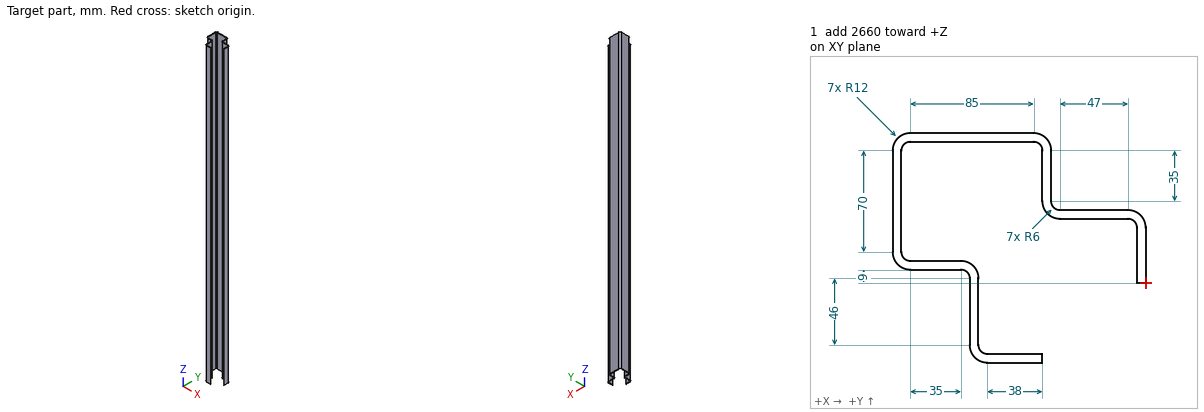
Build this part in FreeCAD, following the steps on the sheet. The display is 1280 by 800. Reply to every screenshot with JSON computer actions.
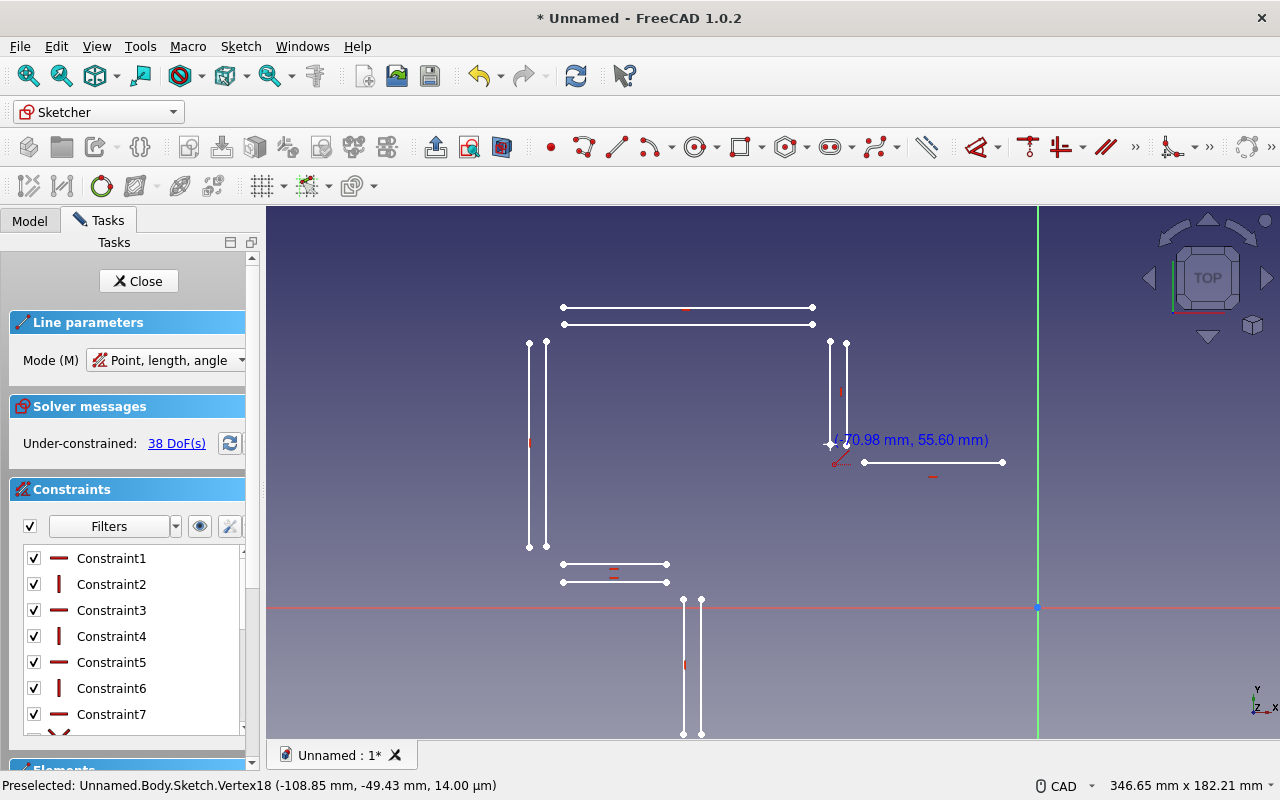
{"action": "left_click", "coordinate": [865, 479]}
{"action": "left_click", "coordinate": [1003, 479]}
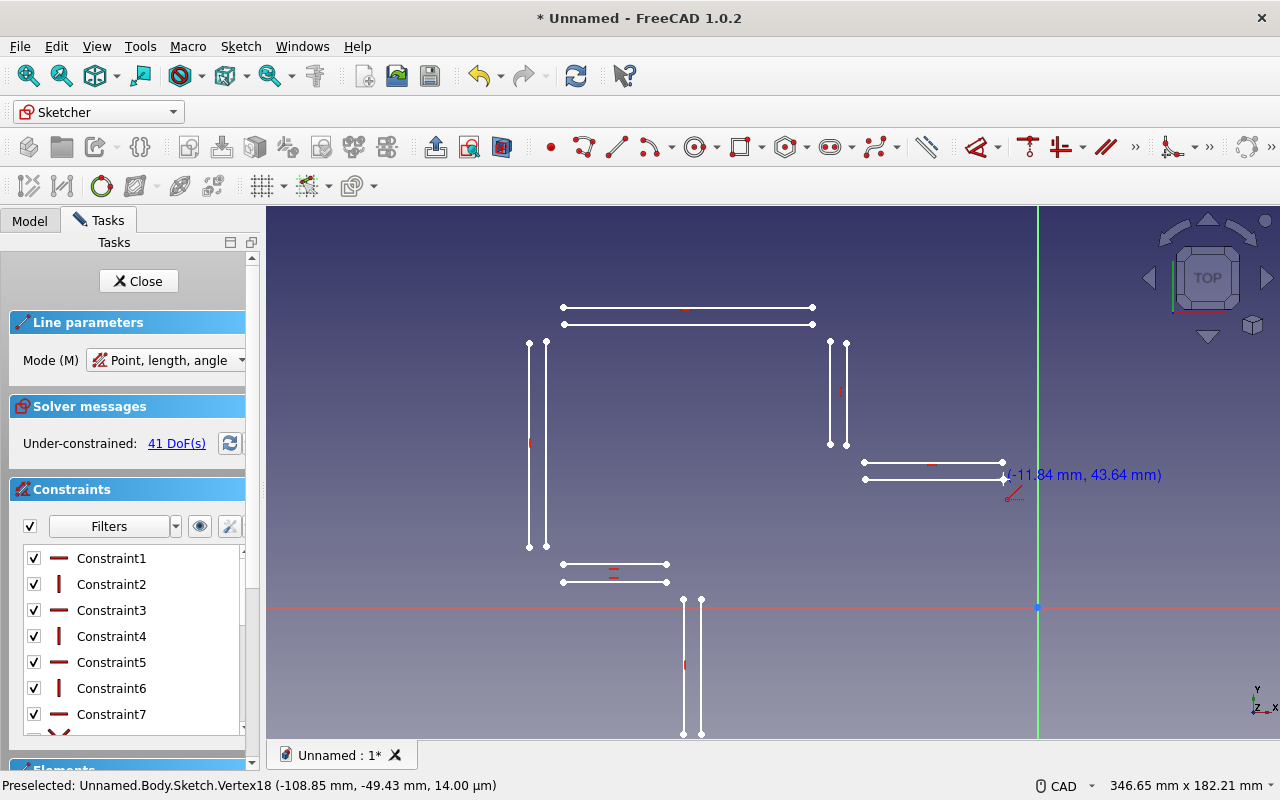
{"action": "key", "text": "g m"}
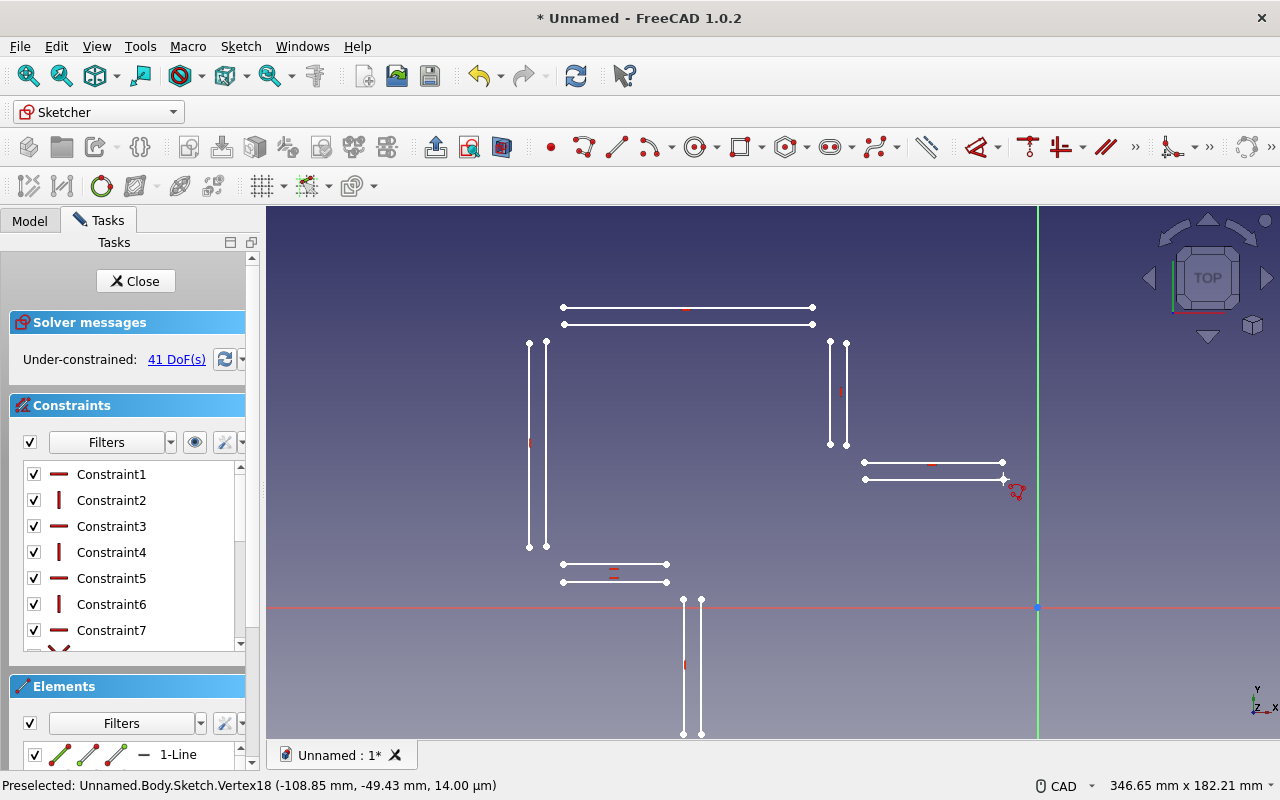
{"action": "left_click", "coordinate": [1020, 496]}
{"action": "left_click", "coordinate": [1020, 608]}
{"action": "left_click", "coordinate": [1038, 608]}
{"action": "left_click", "coordinate": [1029, 496]}
{"action": "right_click", "coordinate": [1029, 496]}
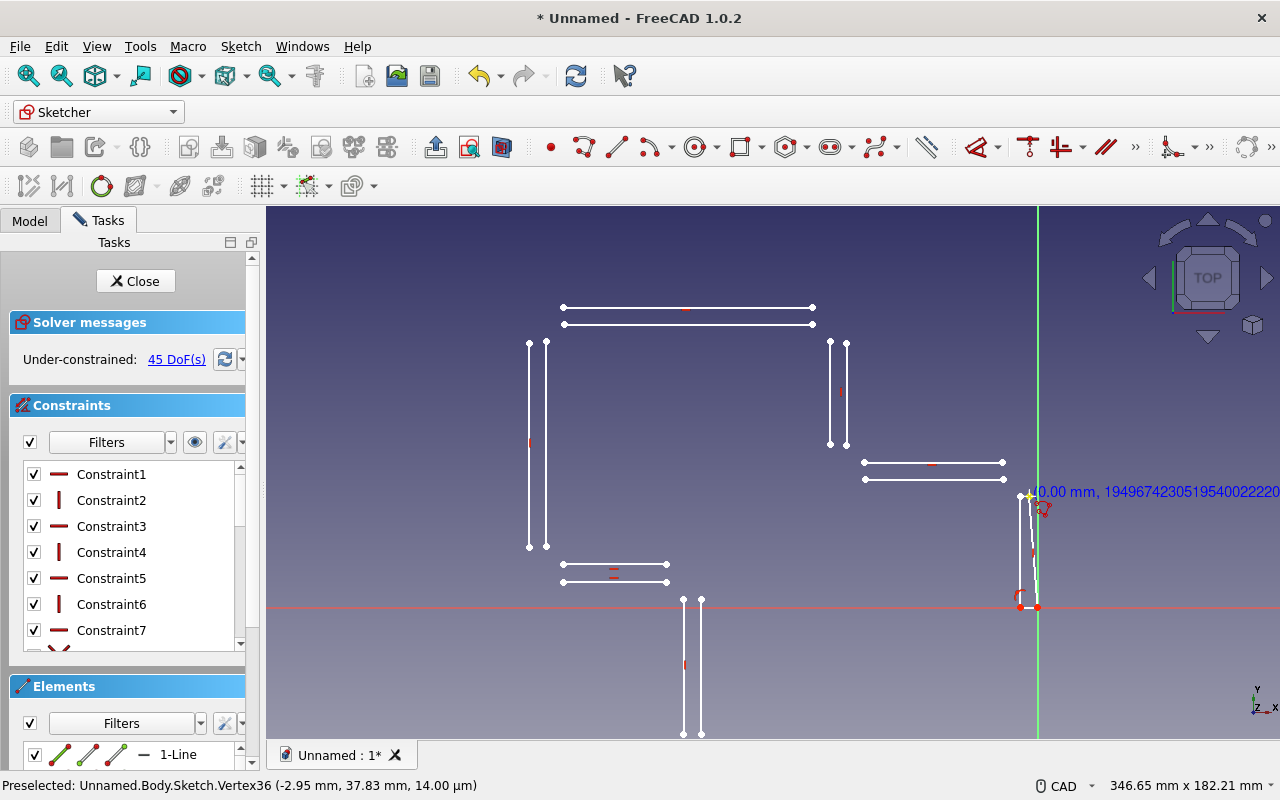
{"action": "key", "text": "g 3 a"}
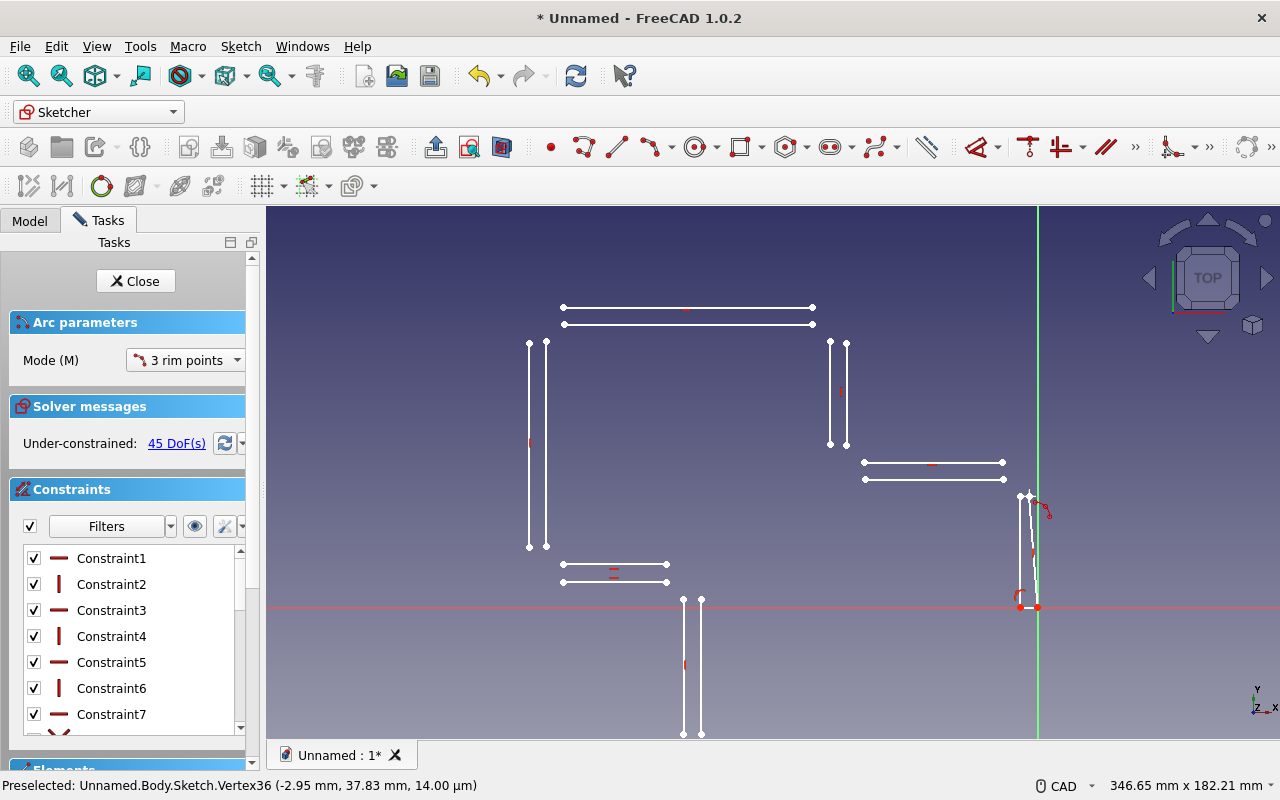
{"action": "left_click", "coordinate": [865, 463]}
{"action": "left_click", "coordinate": [847, 445]}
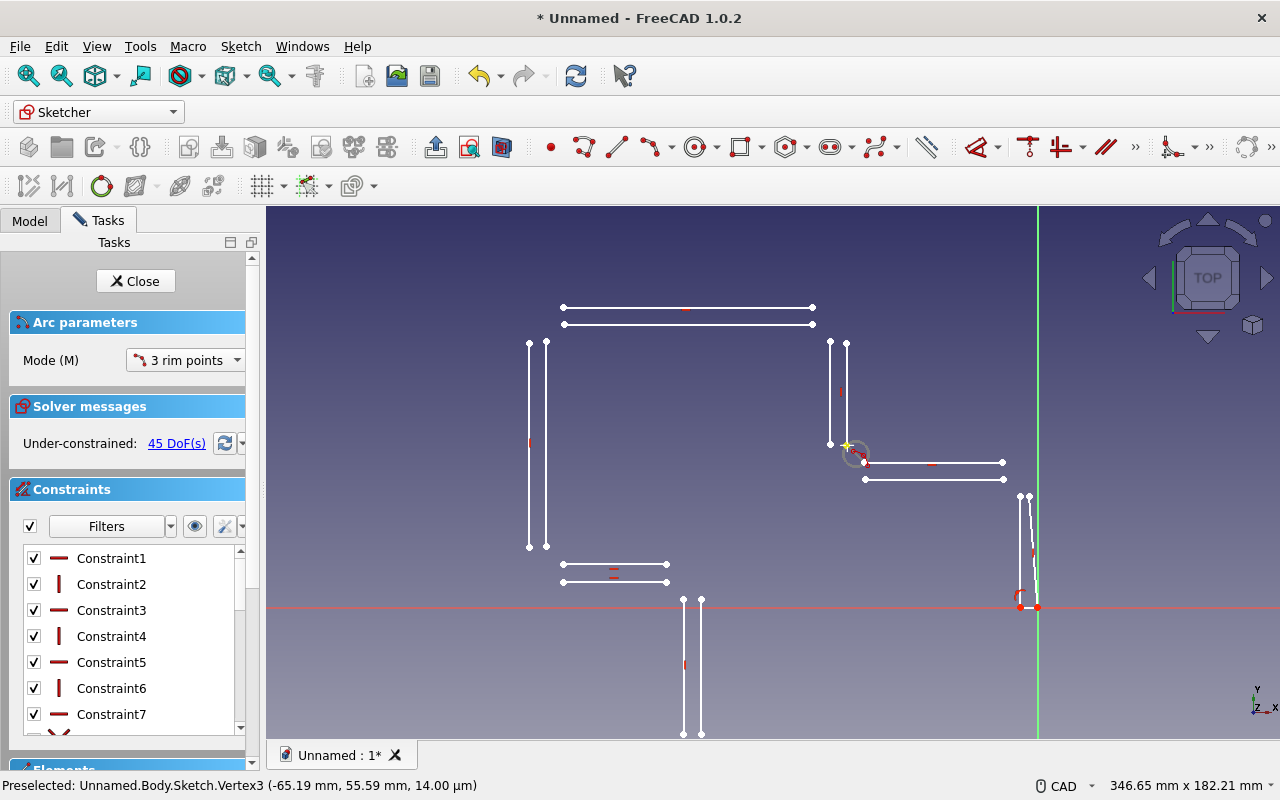
{"action": "scroll", "coordinate": [853, 456], "scroll_direction": "up", "scroll_amount": 6}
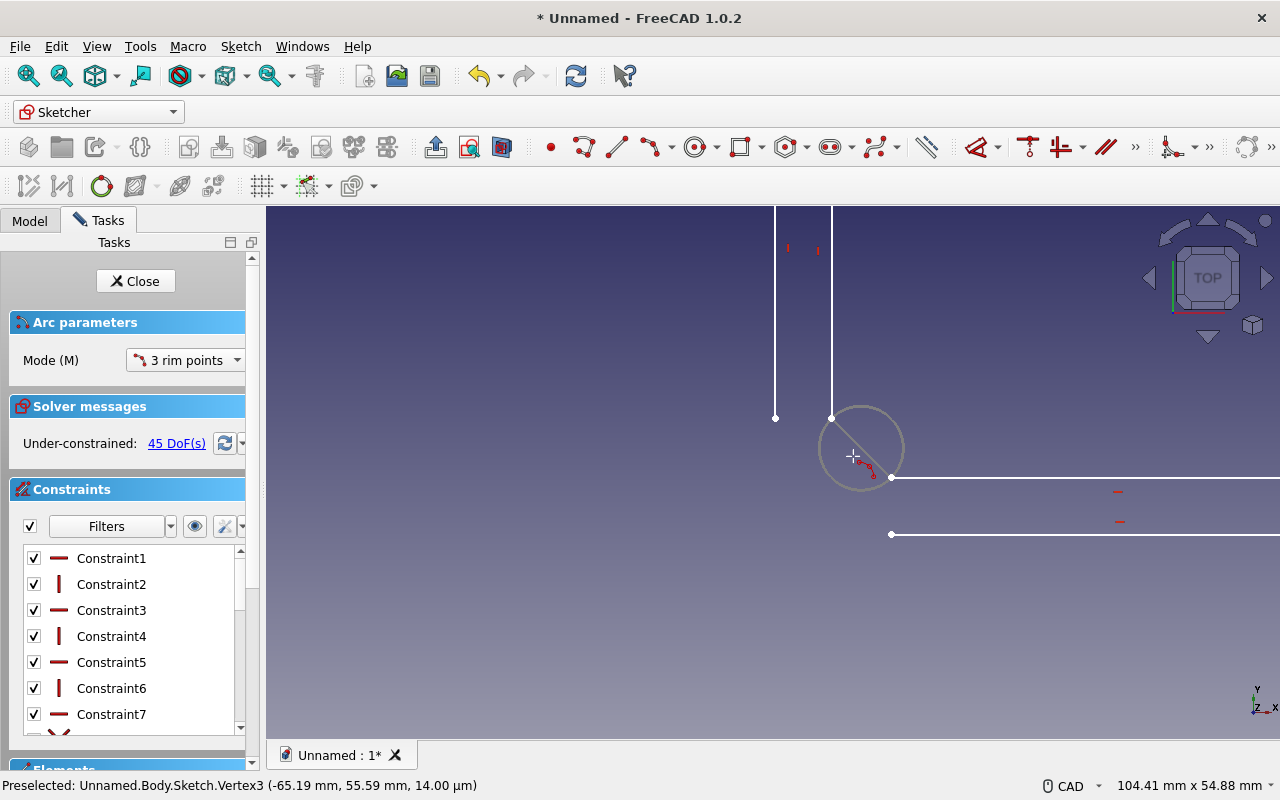
{"action": "left_click", "coordinate": [850, 456]}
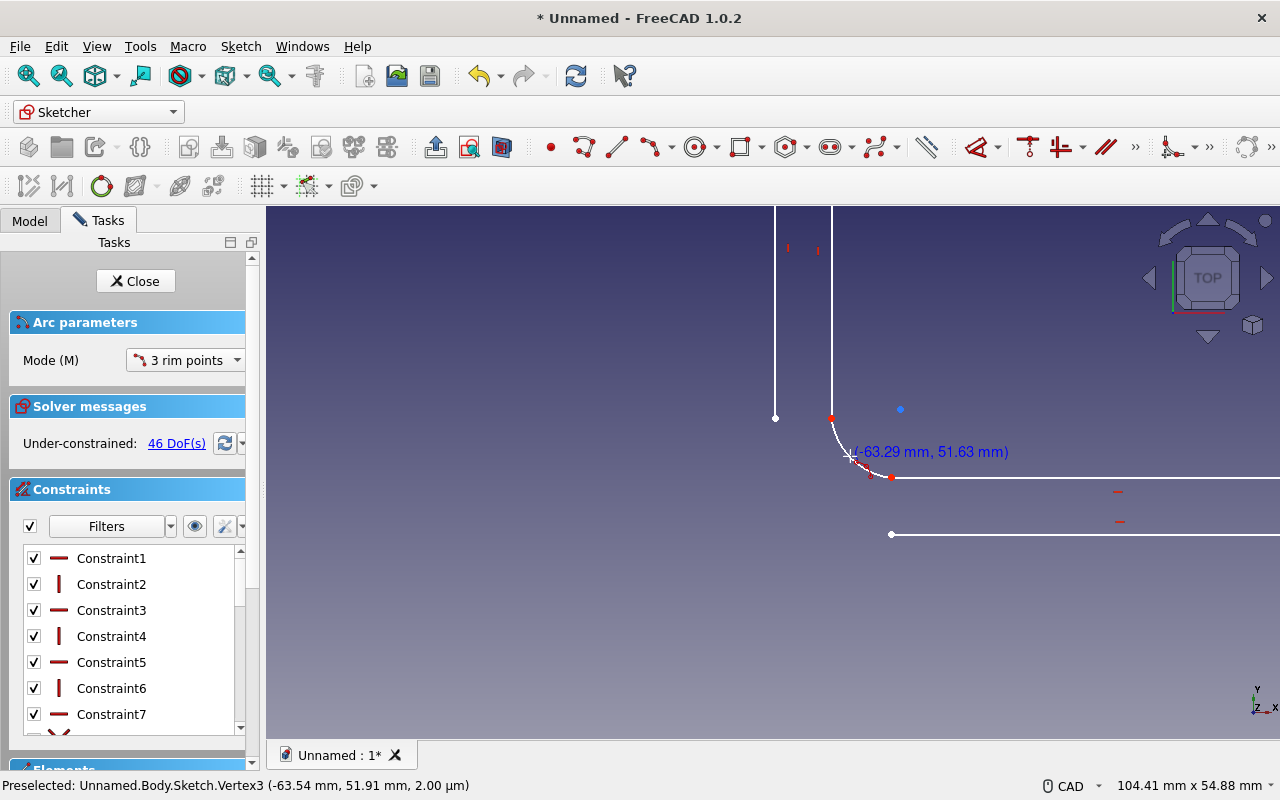
{"action": "scroll", "coordinate": [726, 409], "scroll_direction": "down", "scroll_amount": 8}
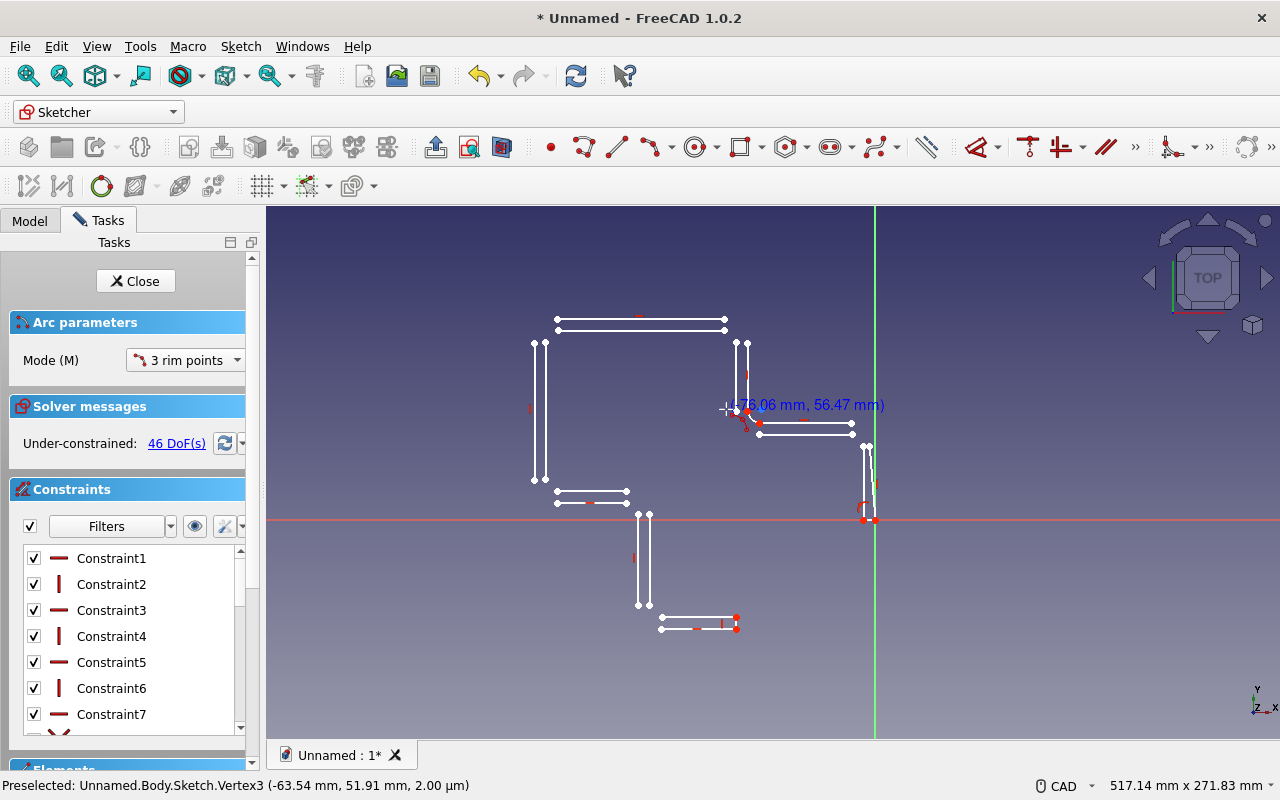
{"action": "scroll", "coordinate": [748, 342], "scroll_direction": "up", "scroll_amount": 2}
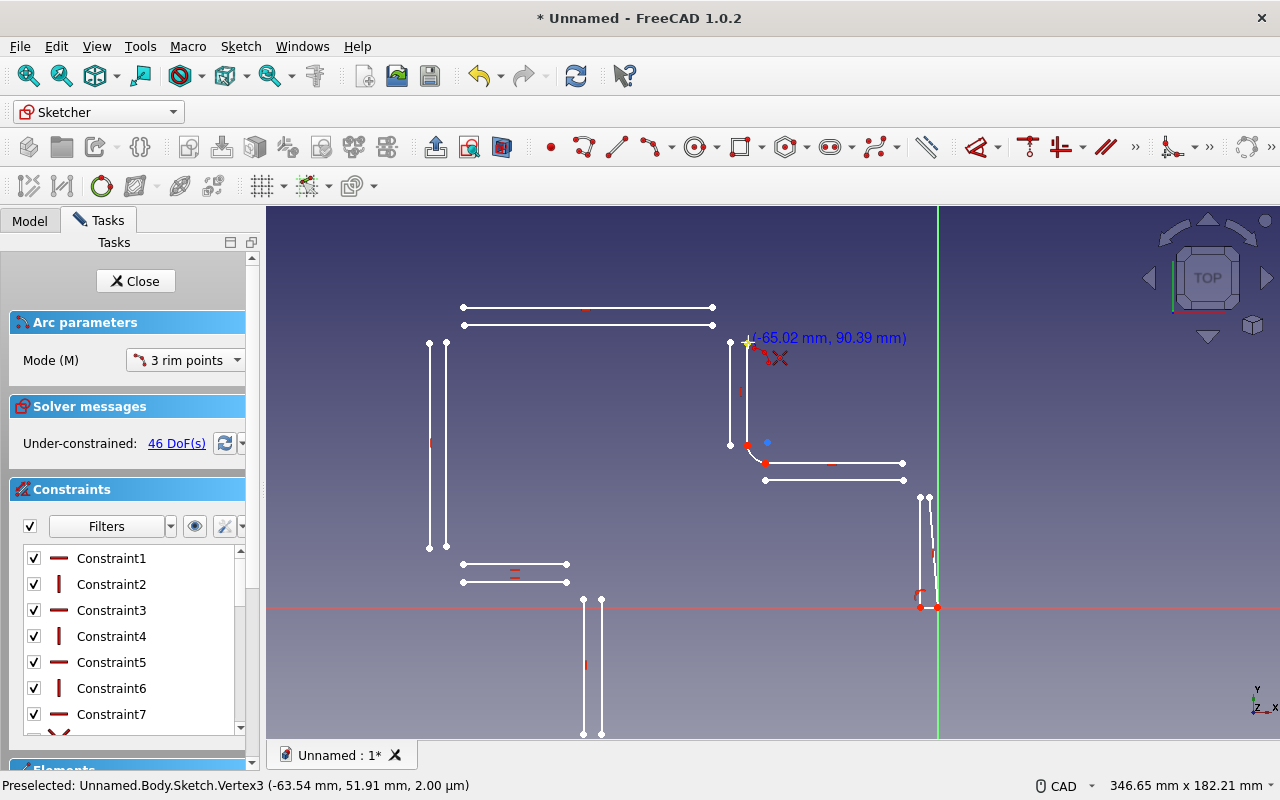
{"action": "left_click", "coordinate": [747, 344]}
{"action": "left_click", "coordinate": [713, 308]}